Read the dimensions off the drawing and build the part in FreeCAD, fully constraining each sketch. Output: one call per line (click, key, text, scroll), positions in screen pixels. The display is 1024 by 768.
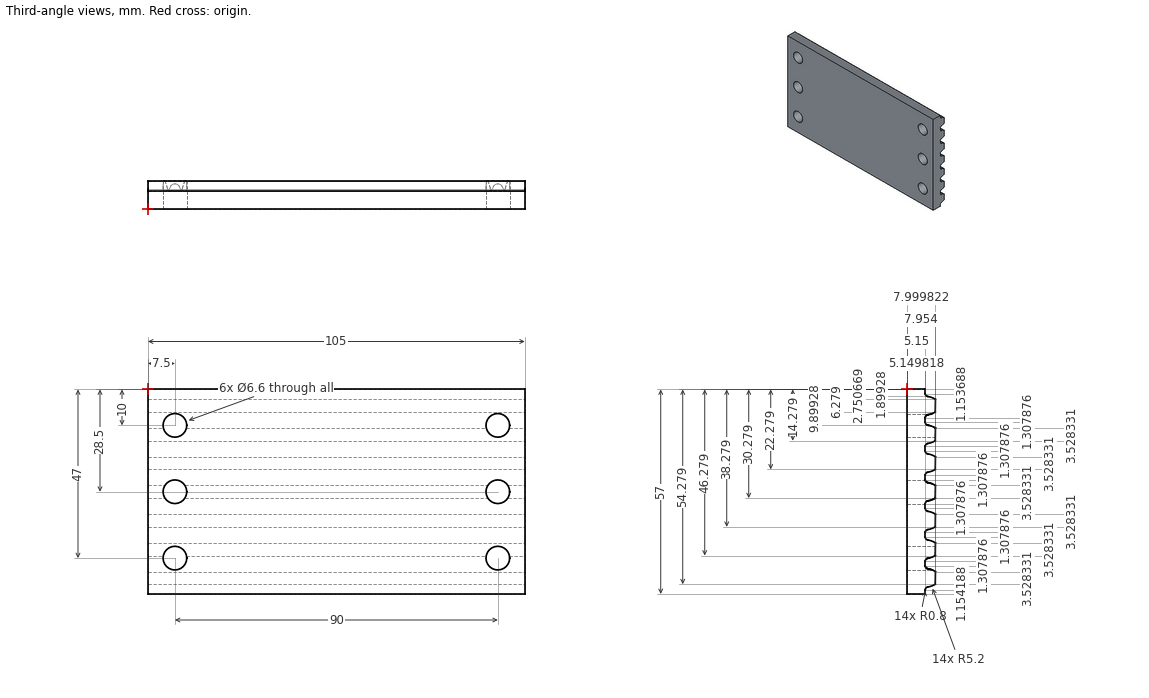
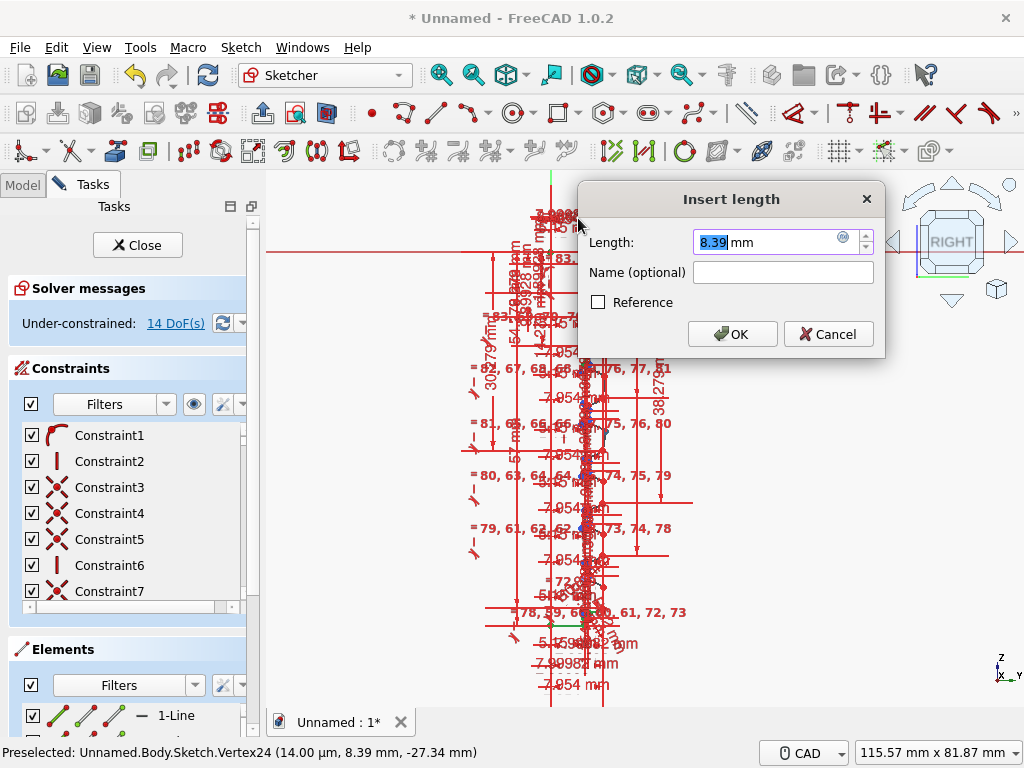
text(7.999822)
key(Return)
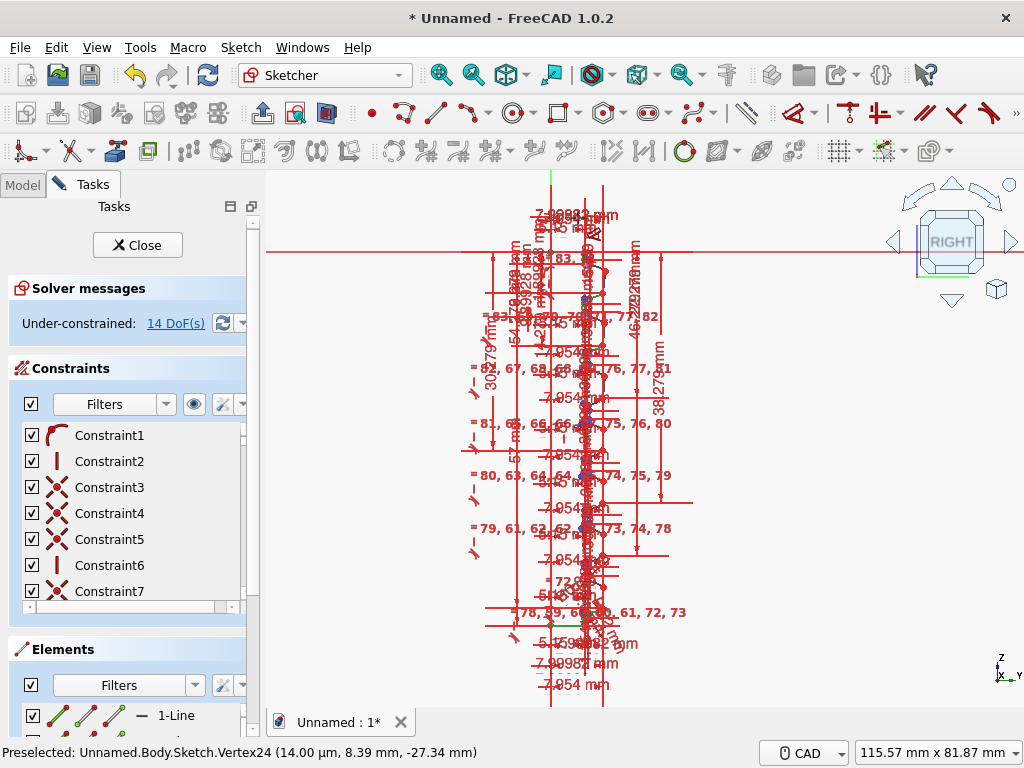
click(605, 377)
click(578, 435)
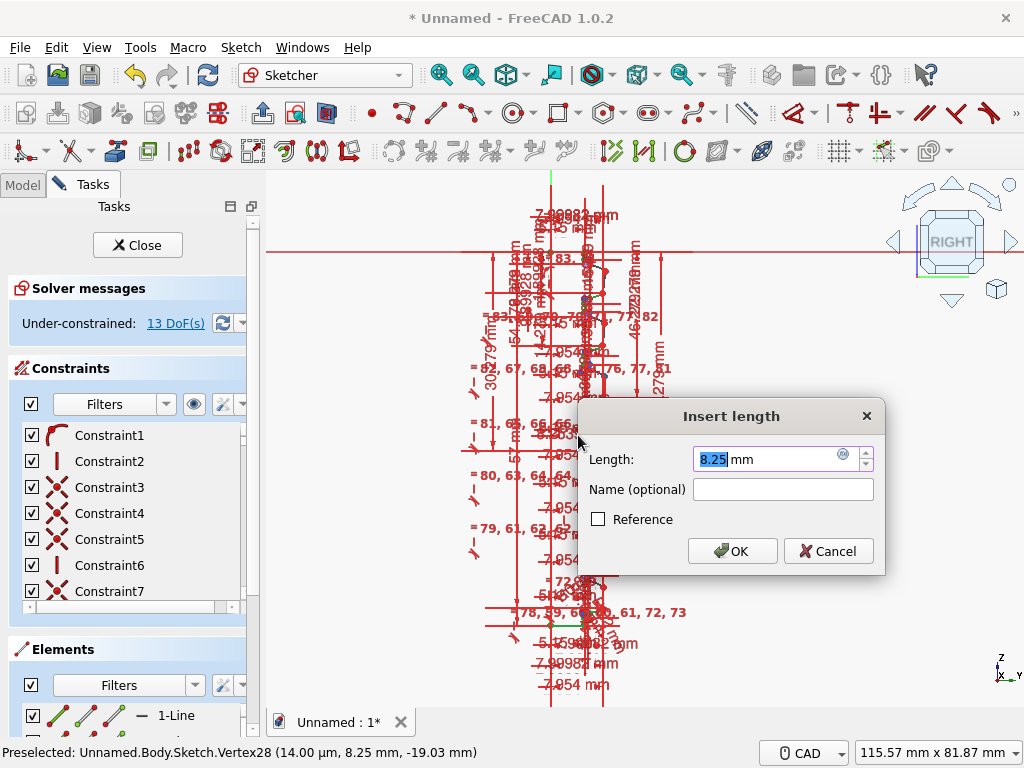
text(7.999822)
key(Return)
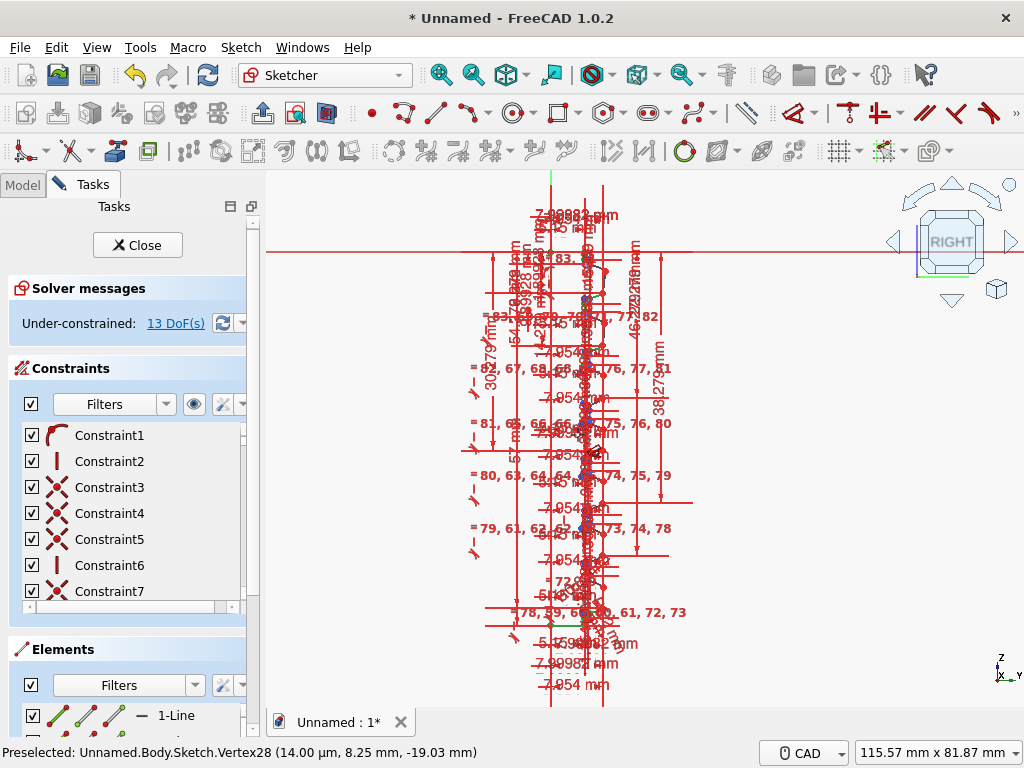
click(605, 323)
click(578, 218)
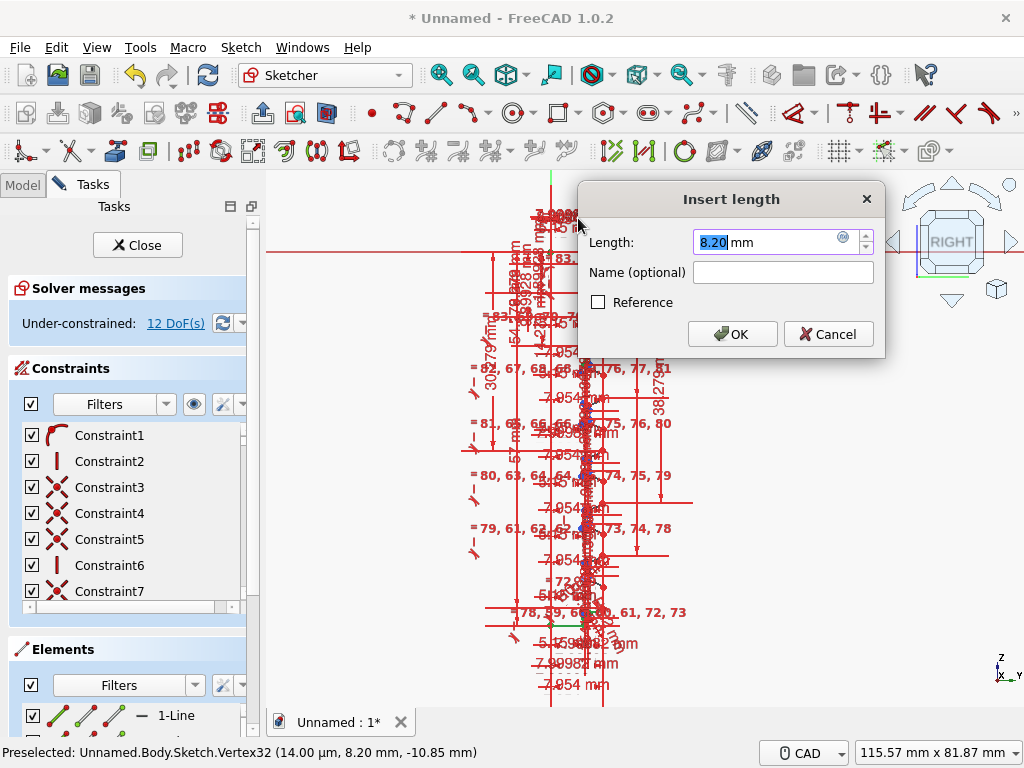
text(7.999822)
key(Return)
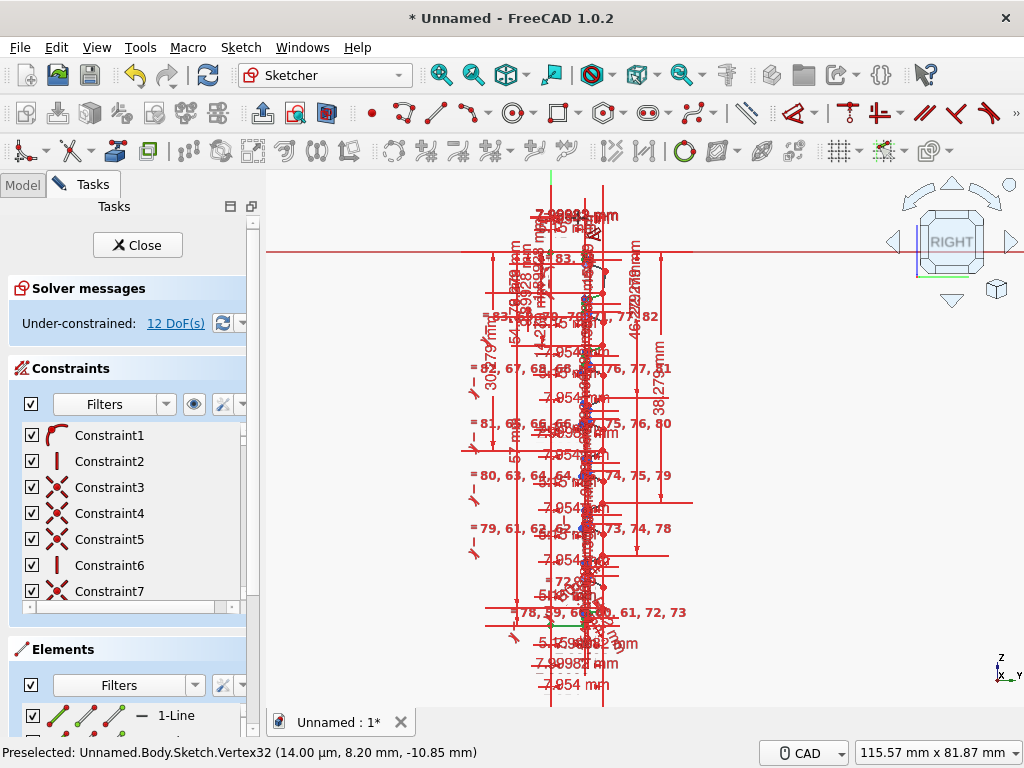
click(605, 271)
click(578, 401)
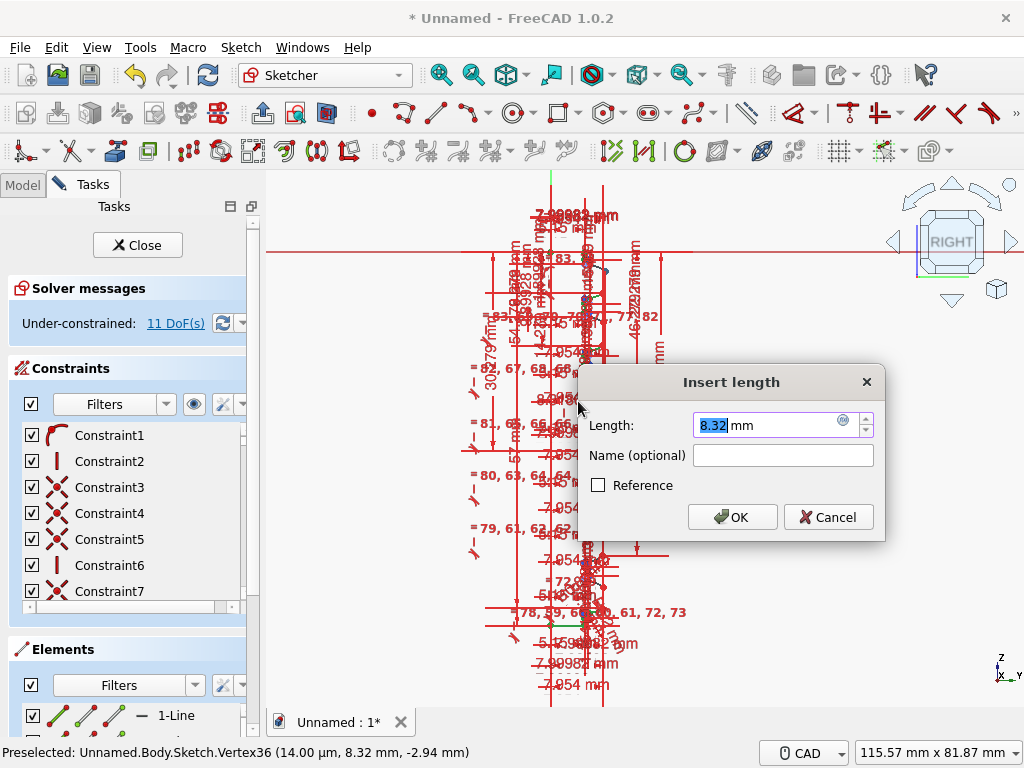
text(7.999822)
key(Return)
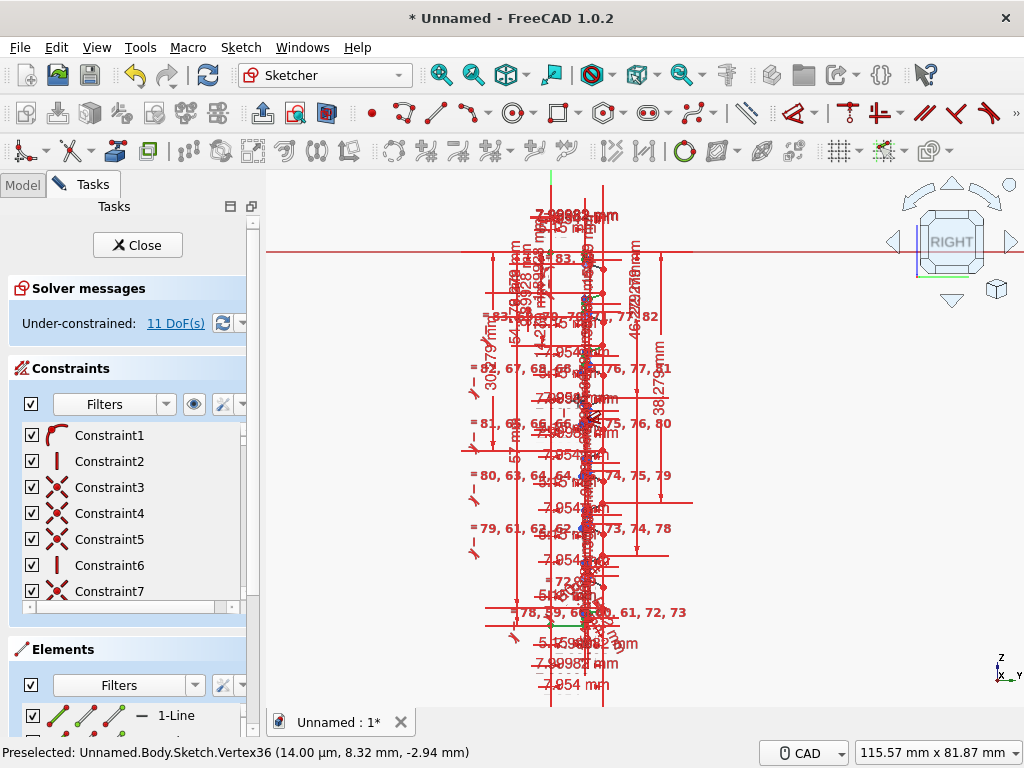
scroll(603, 270, up, 4)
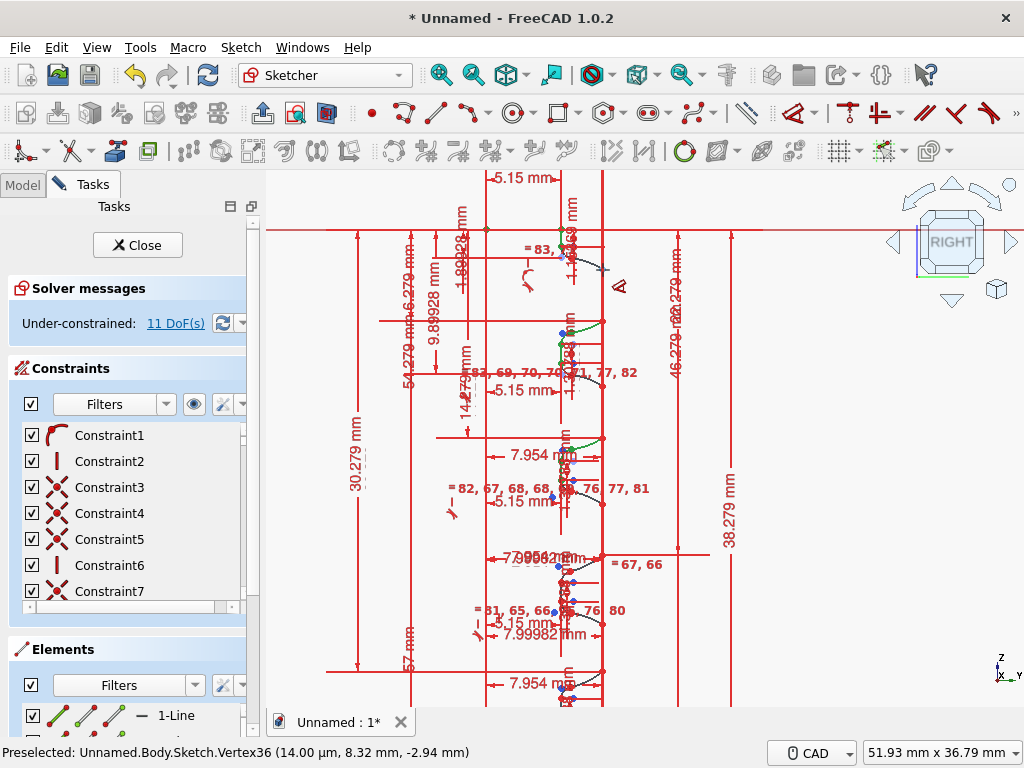
click(603, 270)
click(661, 250)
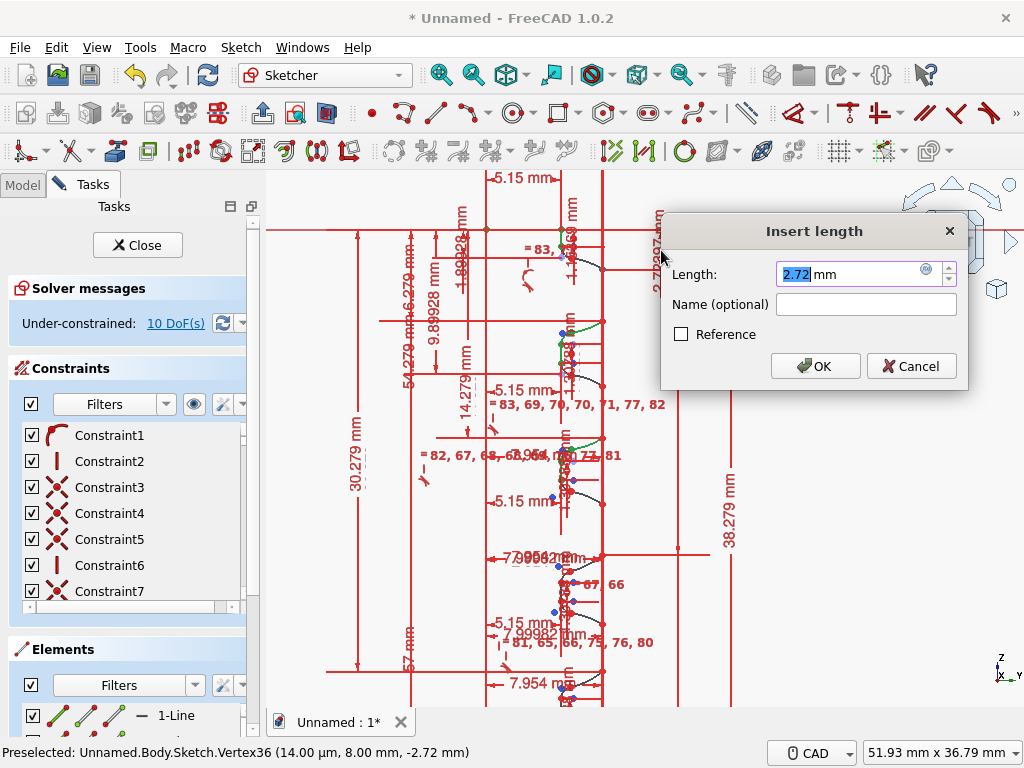
text(2.750669)
key(Return)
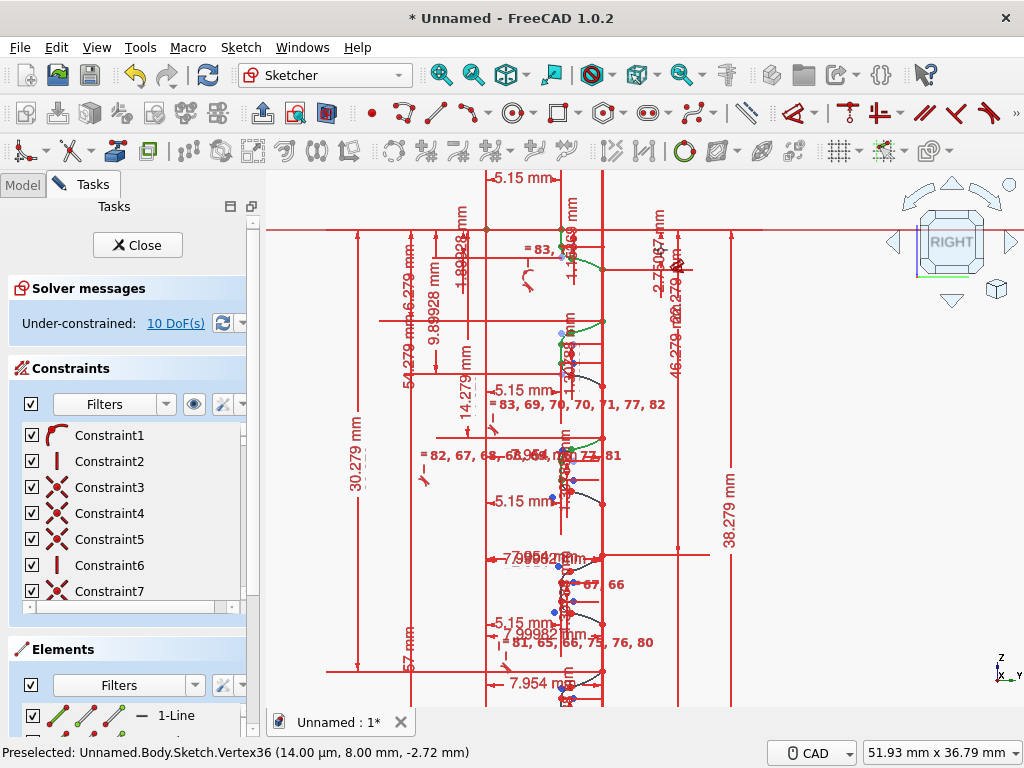
scroll(603, 269, down, 4)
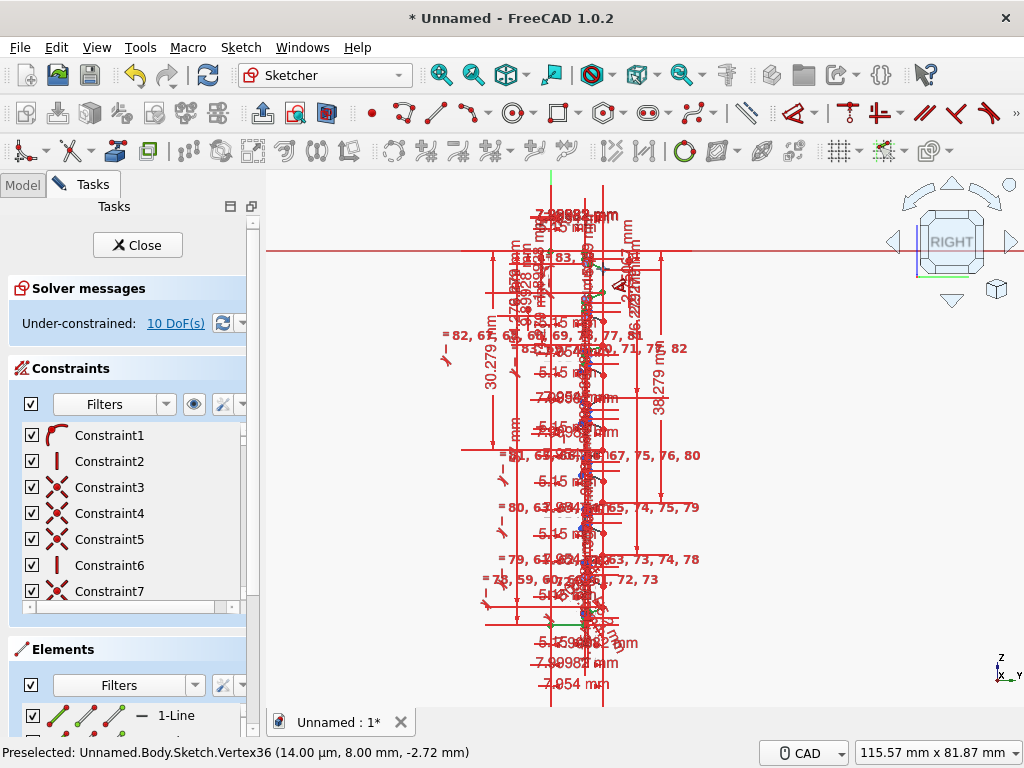
scroll(603, 601, up, 4)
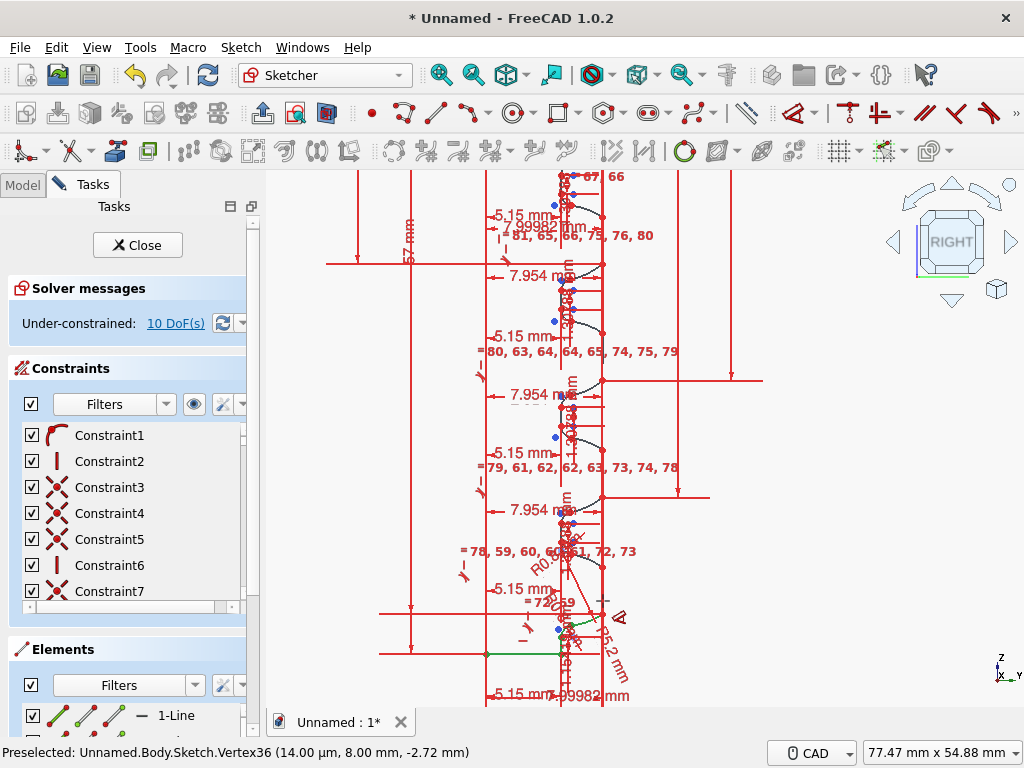
click(602, 600)
click(637, 591)